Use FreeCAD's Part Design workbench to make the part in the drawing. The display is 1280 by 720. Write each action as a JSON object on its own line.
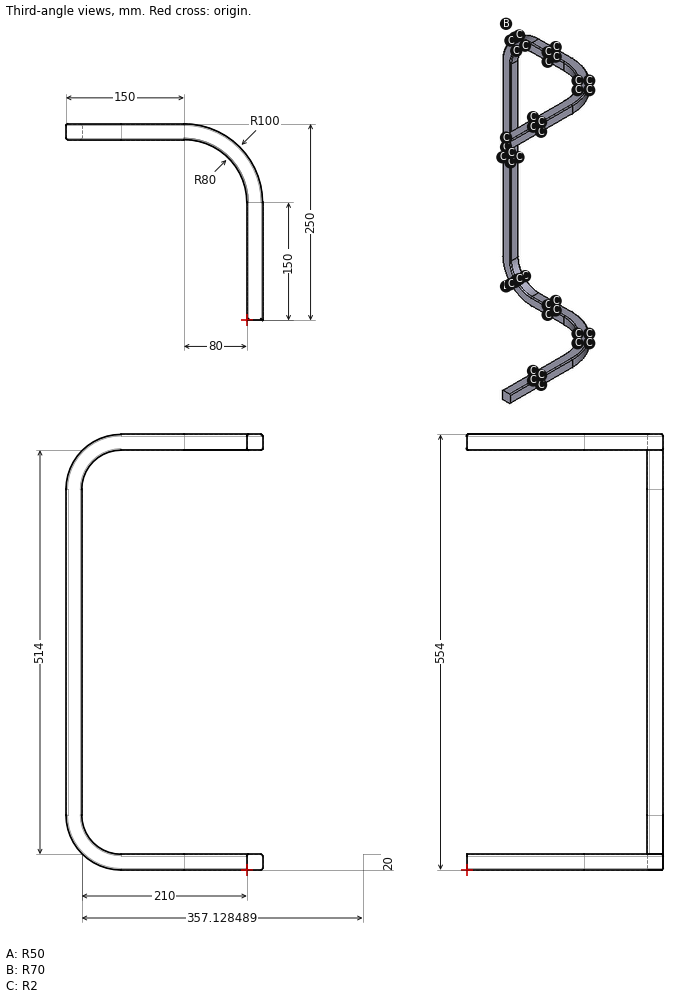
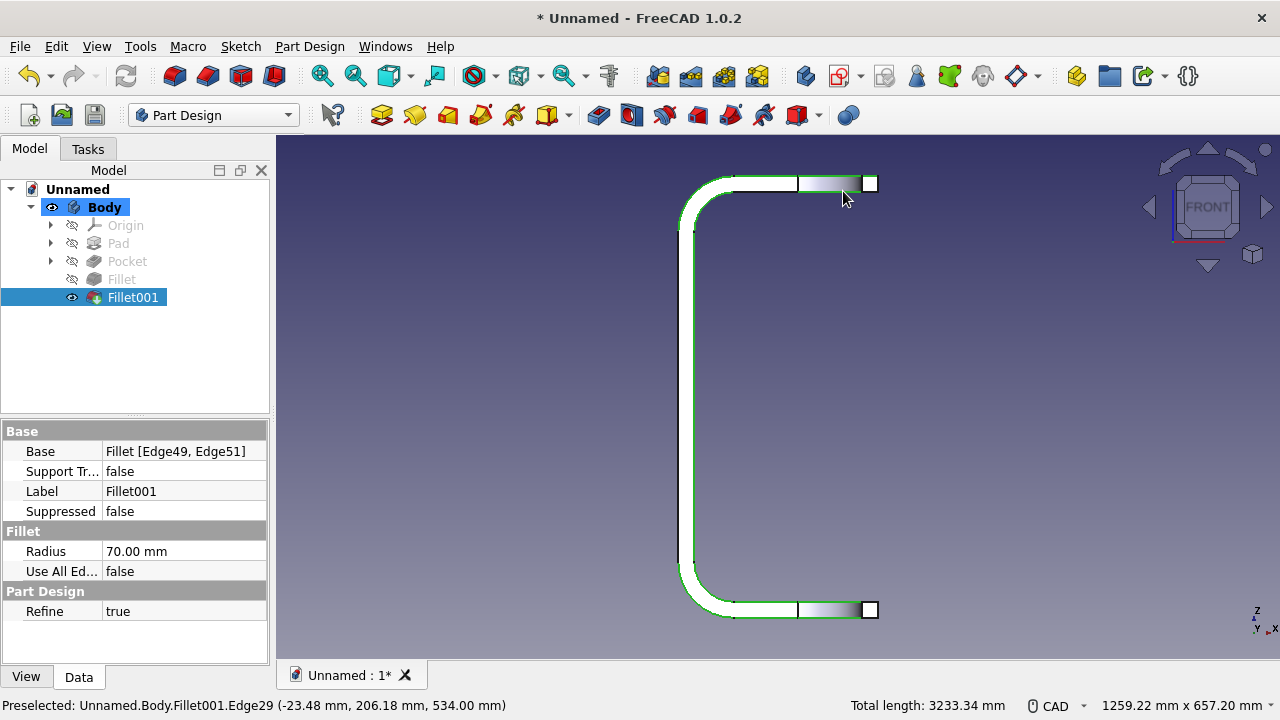
{"action": "left_click", "coordinate": [870, 191], "text": "ctrl"}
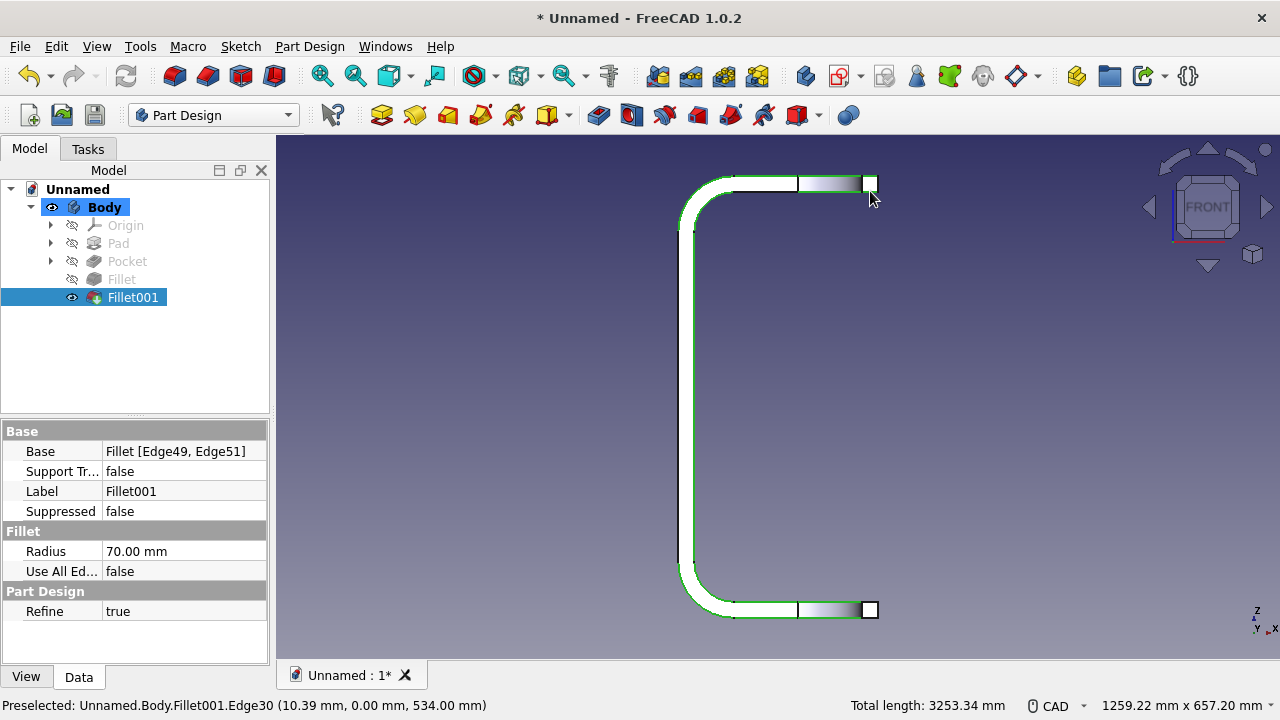
{"action": "left_click", "coordinate": [766, 191], "text": "ctrl"}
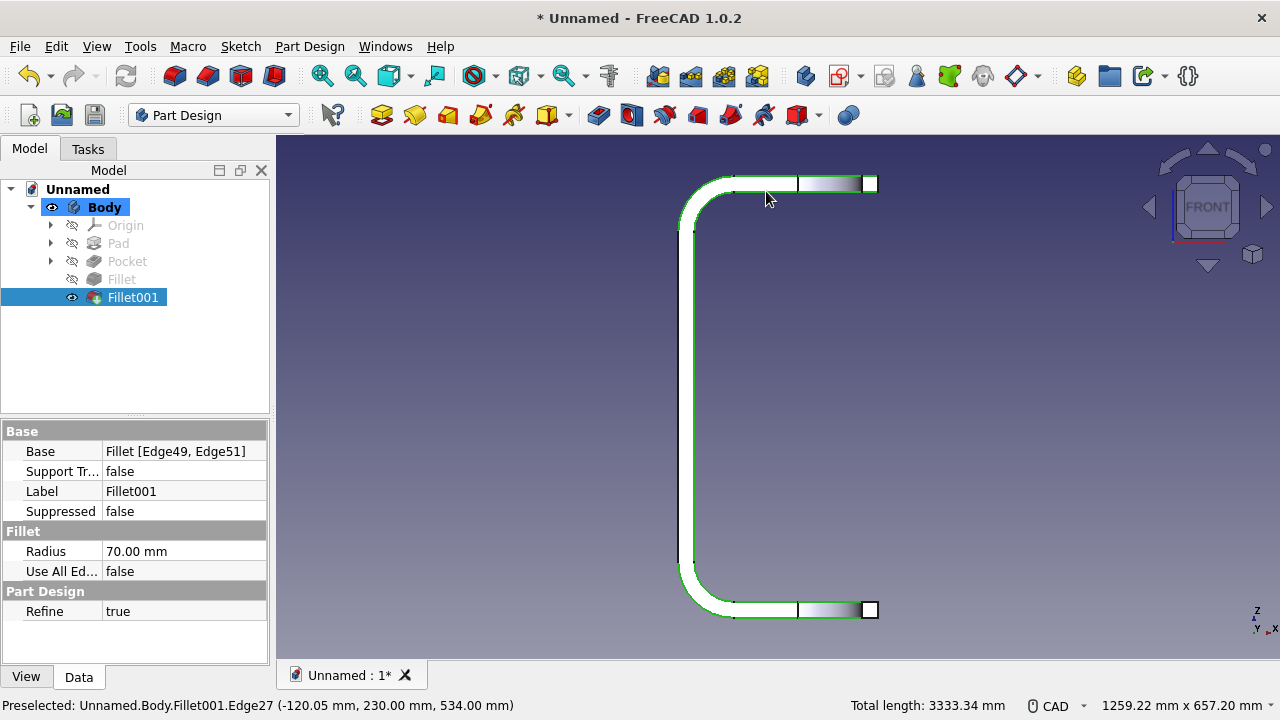
{"action": "left_click", "coordinate": [678, 396], "text": "ctrl"}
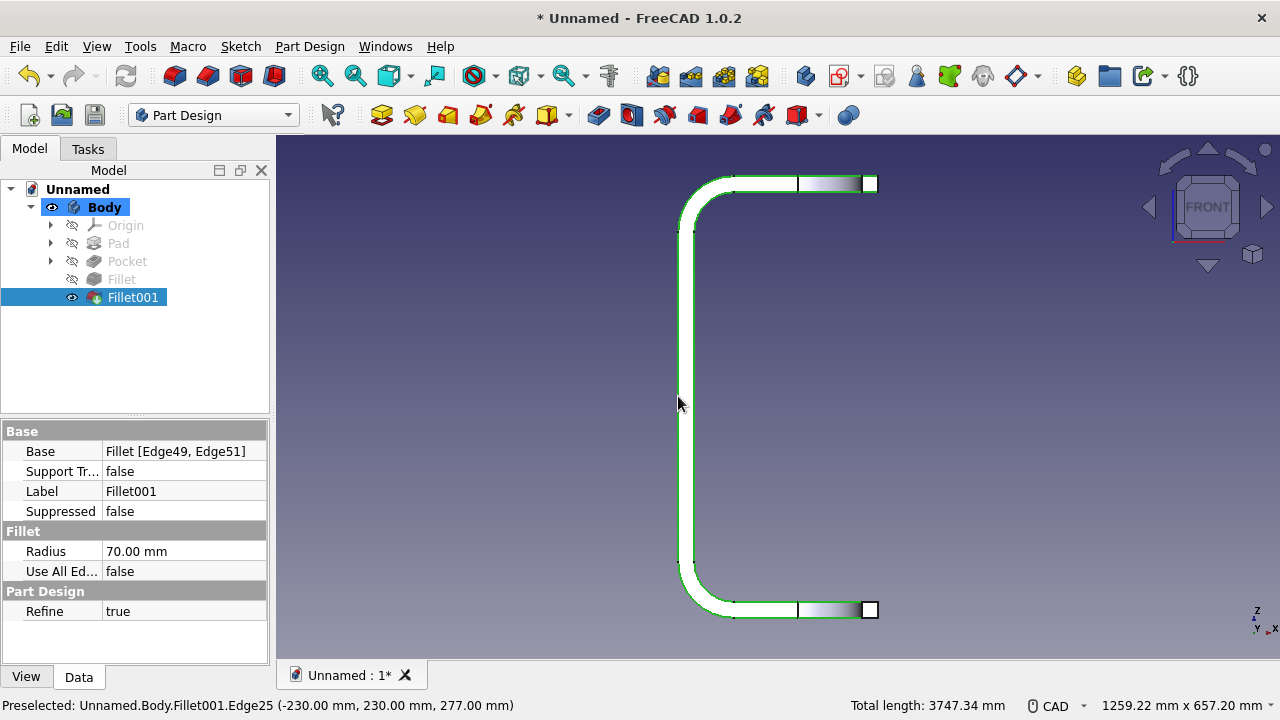
{"action": "key", "text": "3"}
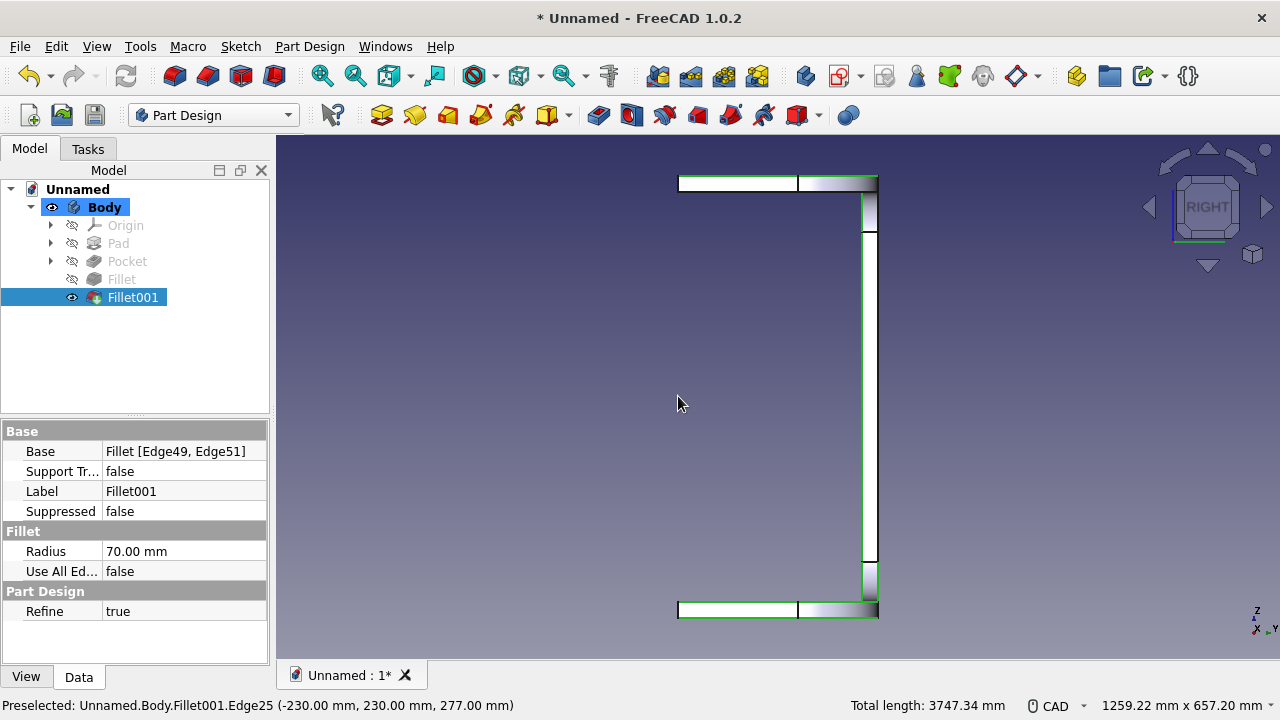
{"action": "left_click", "coordinate": [738, 191], "text": "ctrl"}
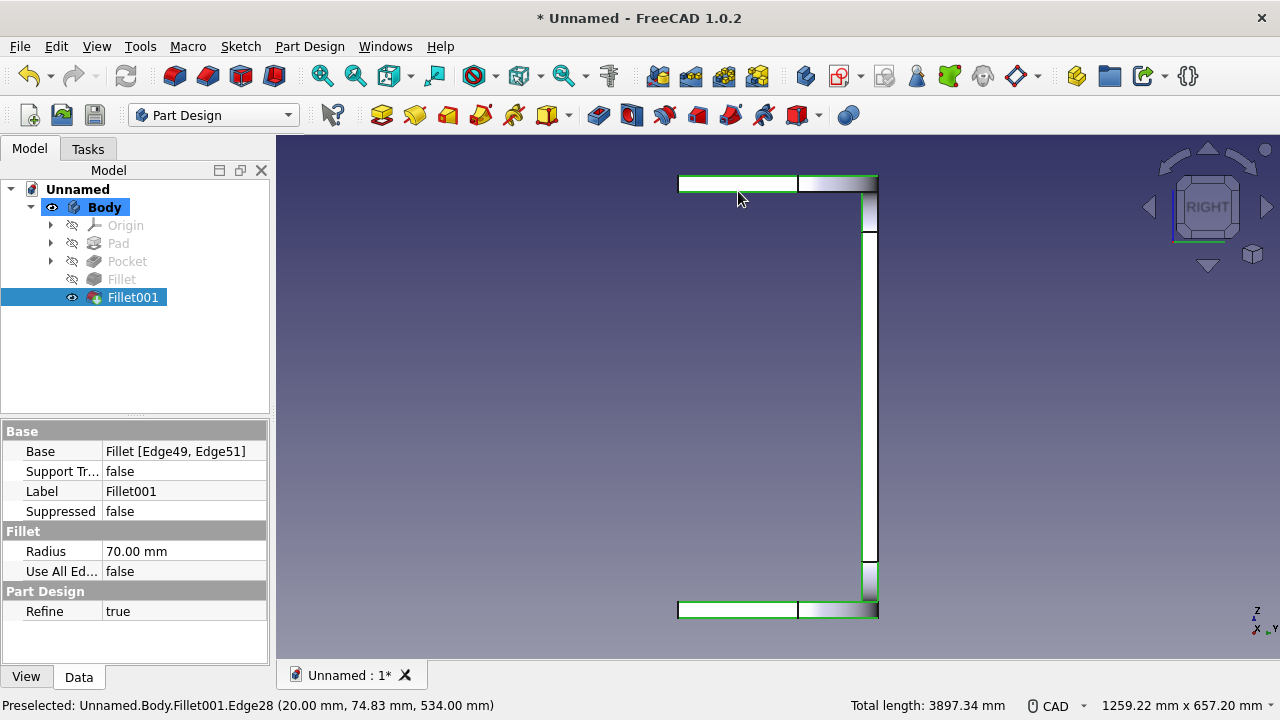
{"action": "left_click", "coordinate": [854, 191], "text": "ctrl"}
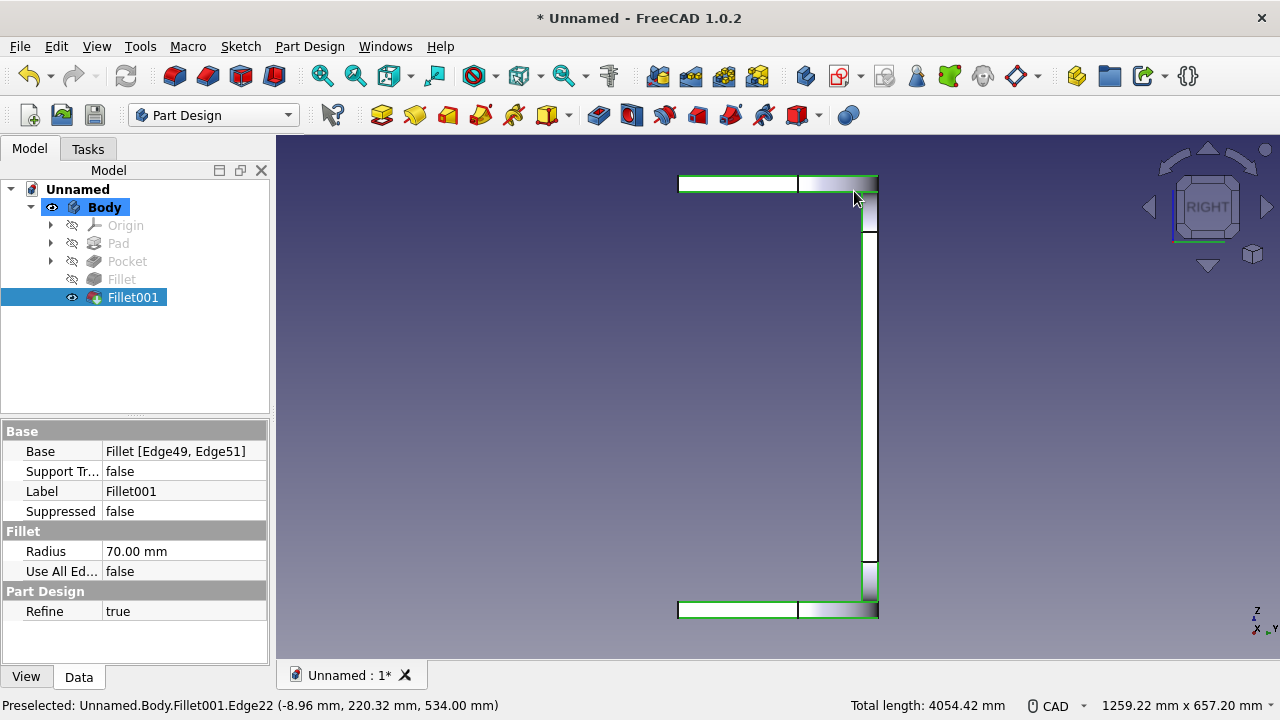
{"action": "left_click", "coordinate": [878, 396], "text": "ctrl"}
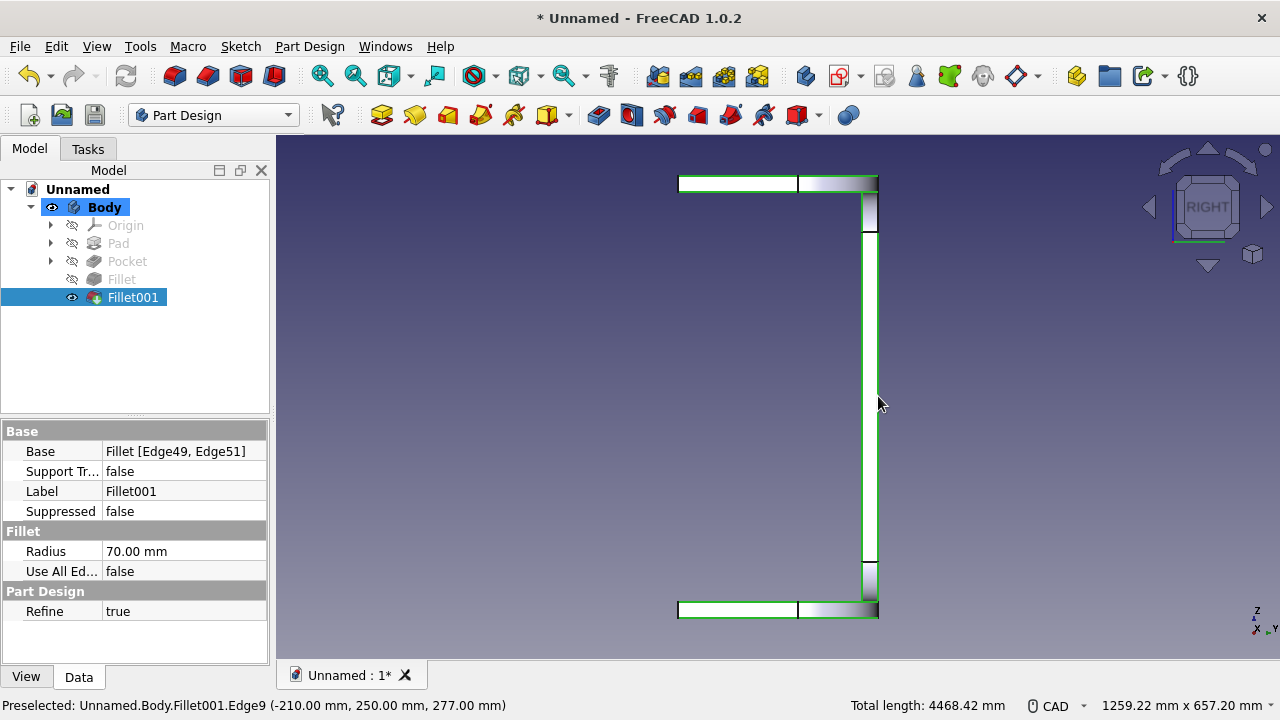
{"action": "left_click", "coordinate": [878, 203], "text": "ctrl"}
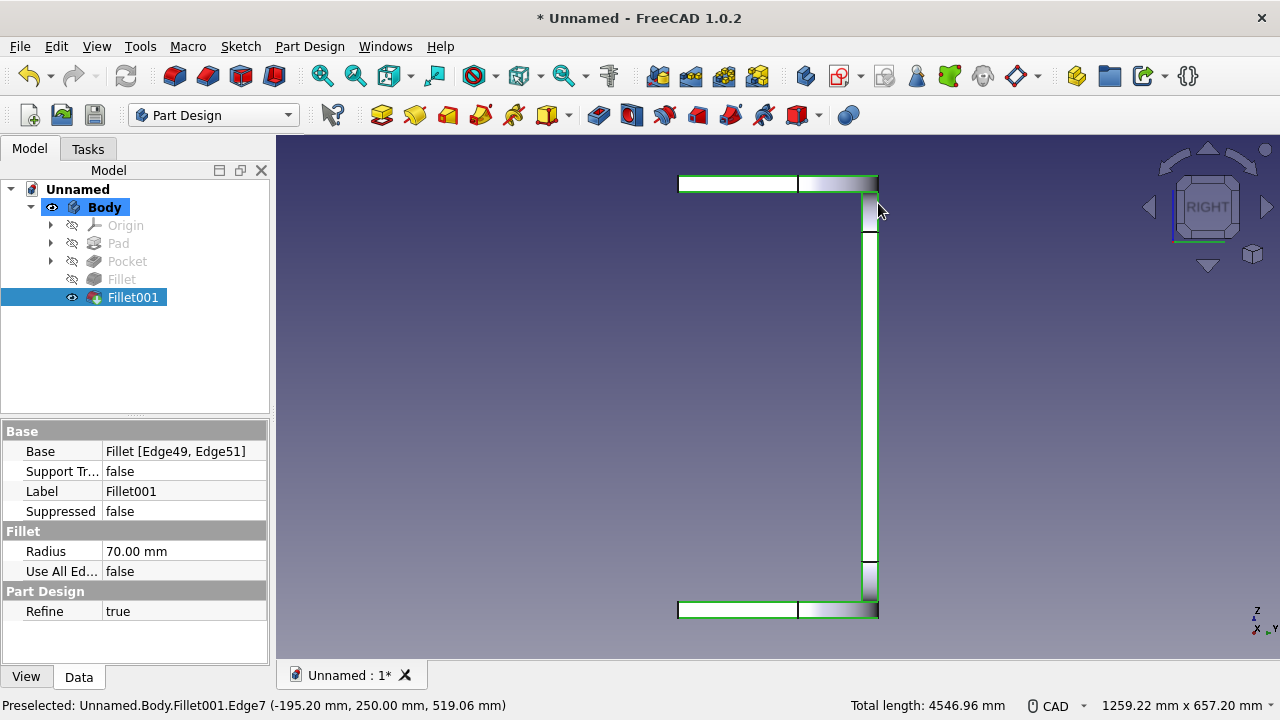
{"action": "key", "text": "5"}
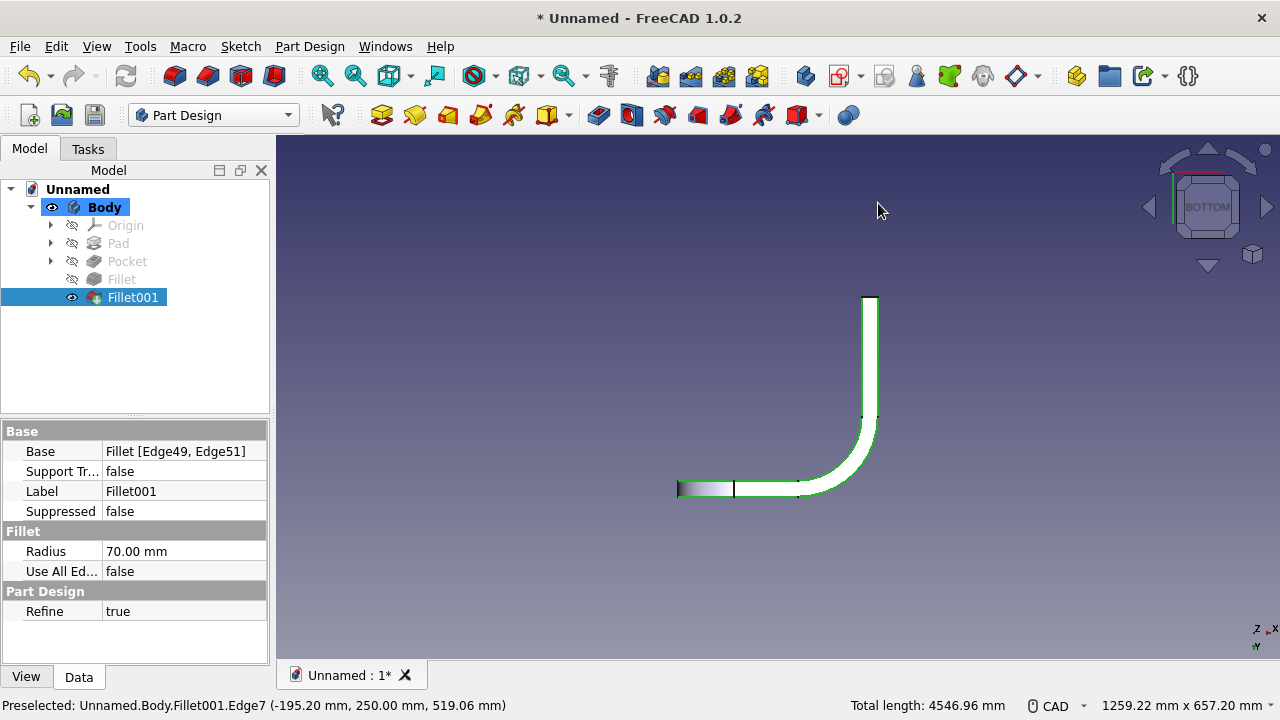
{"action": "left_click", "coordinate": [323, 76]}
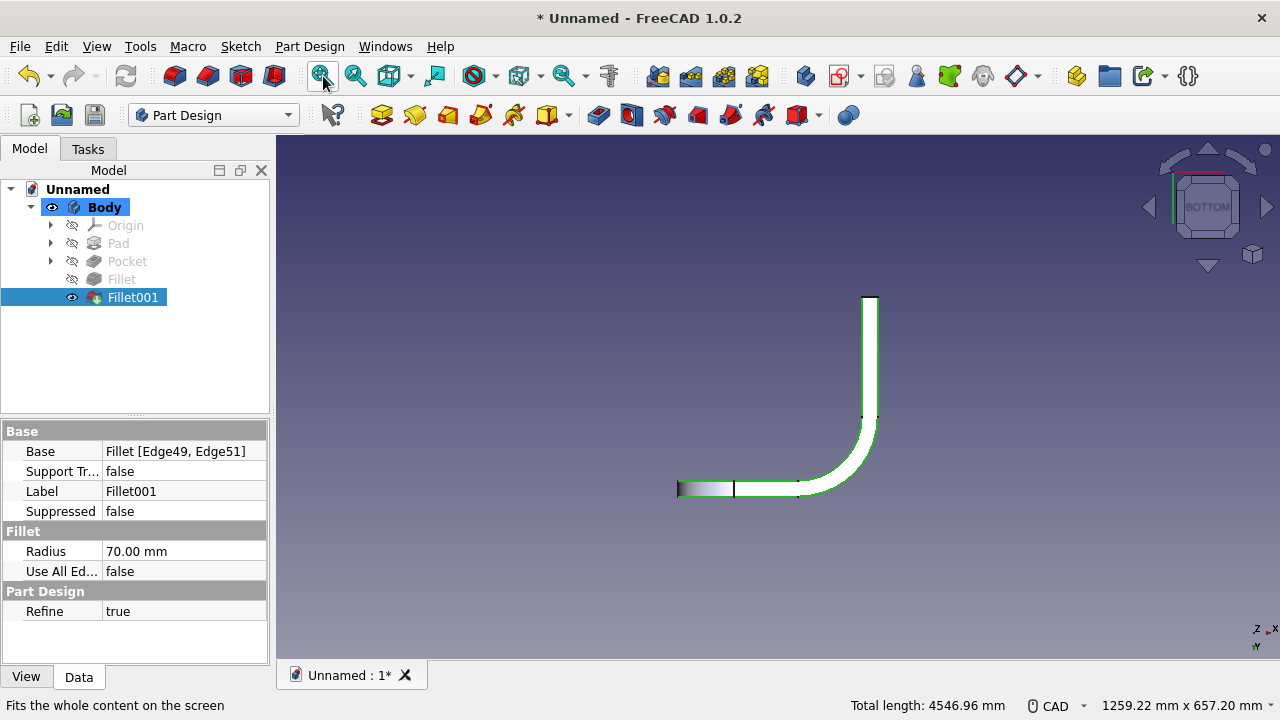
{"action": "key", "text": "4"}